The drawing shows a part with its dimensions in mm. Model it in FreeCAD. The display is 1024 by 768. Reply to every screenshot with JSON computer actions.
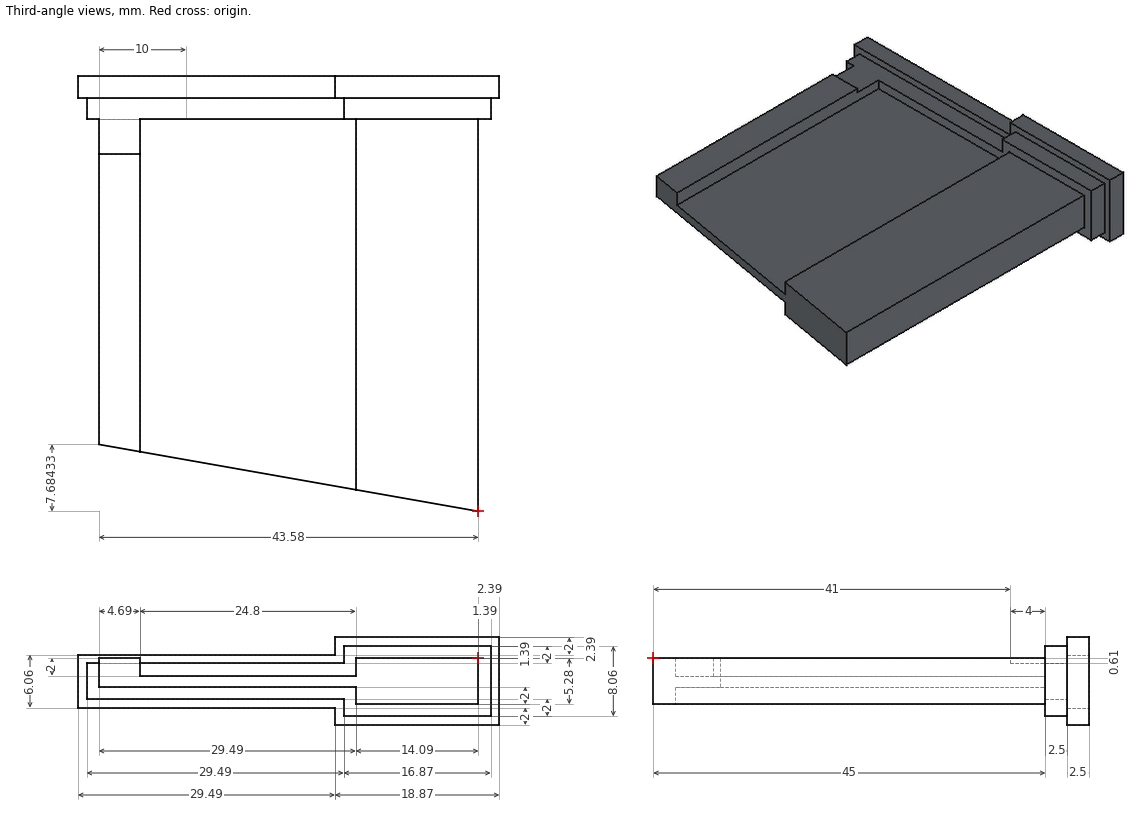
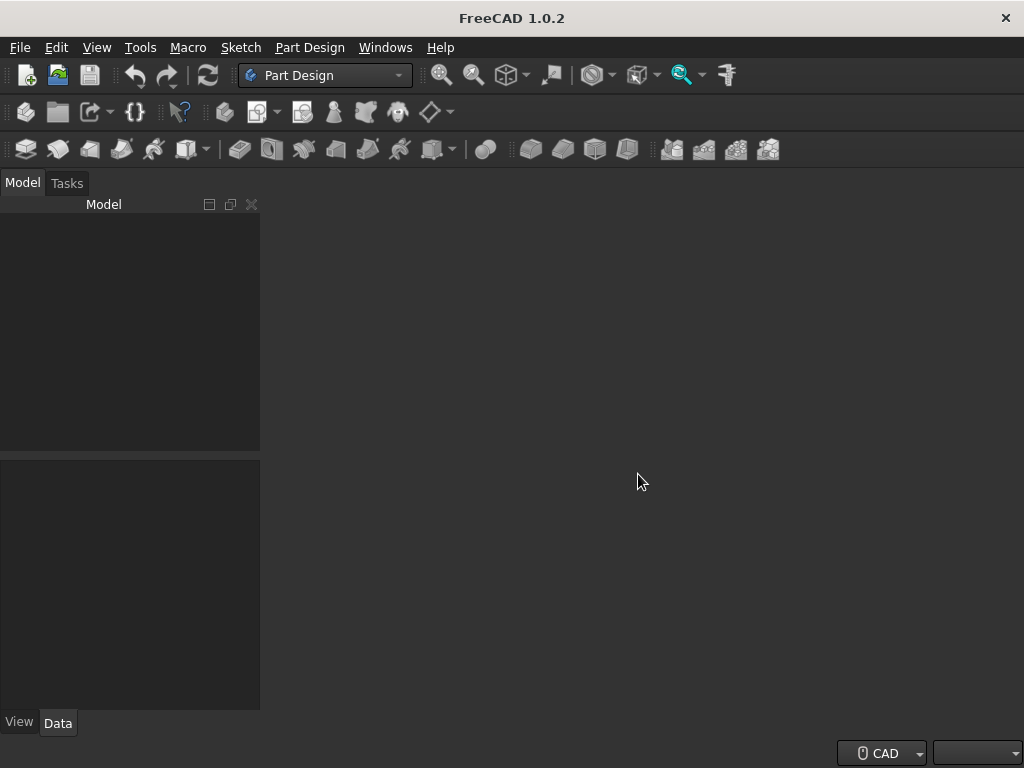
{"action": "left_click", "coordinate": [26, 76]}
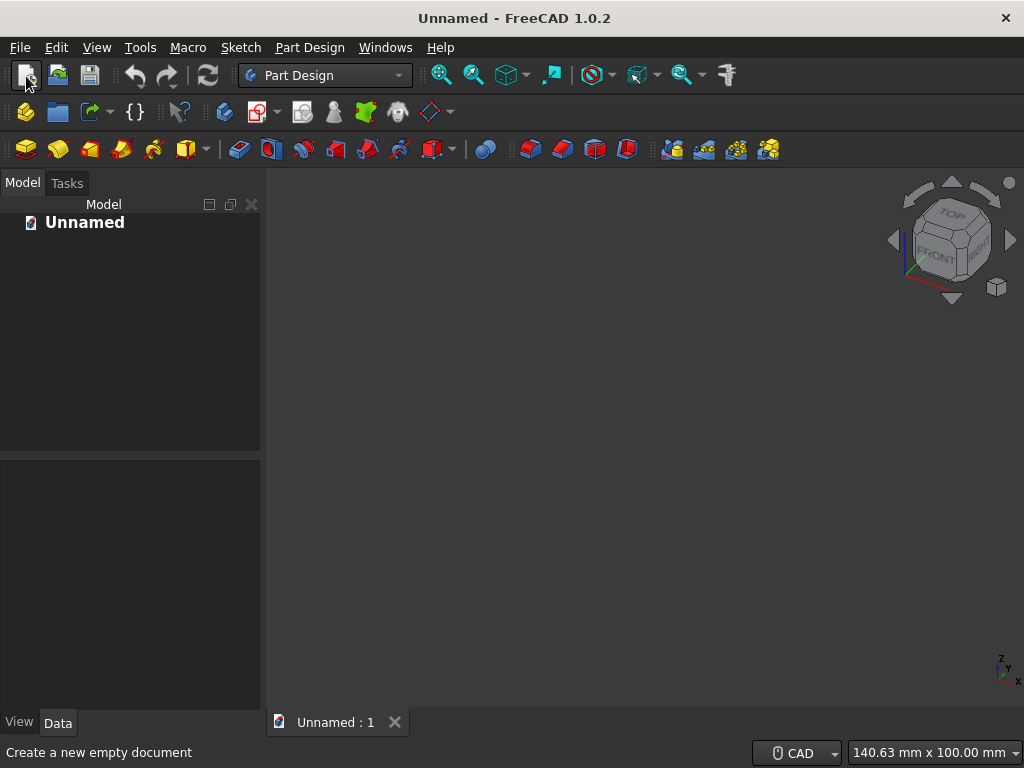
{"action": "left_click", "coordinate": [258, 112]}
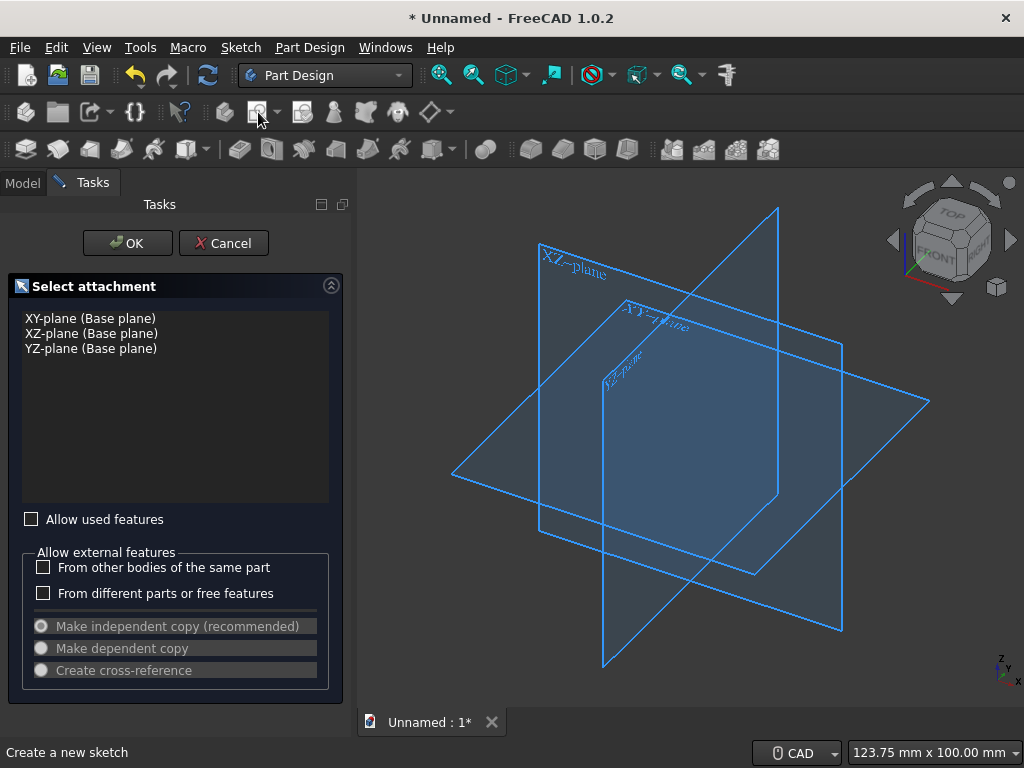
{"action": "left_click", "coordinate": [82, 334]}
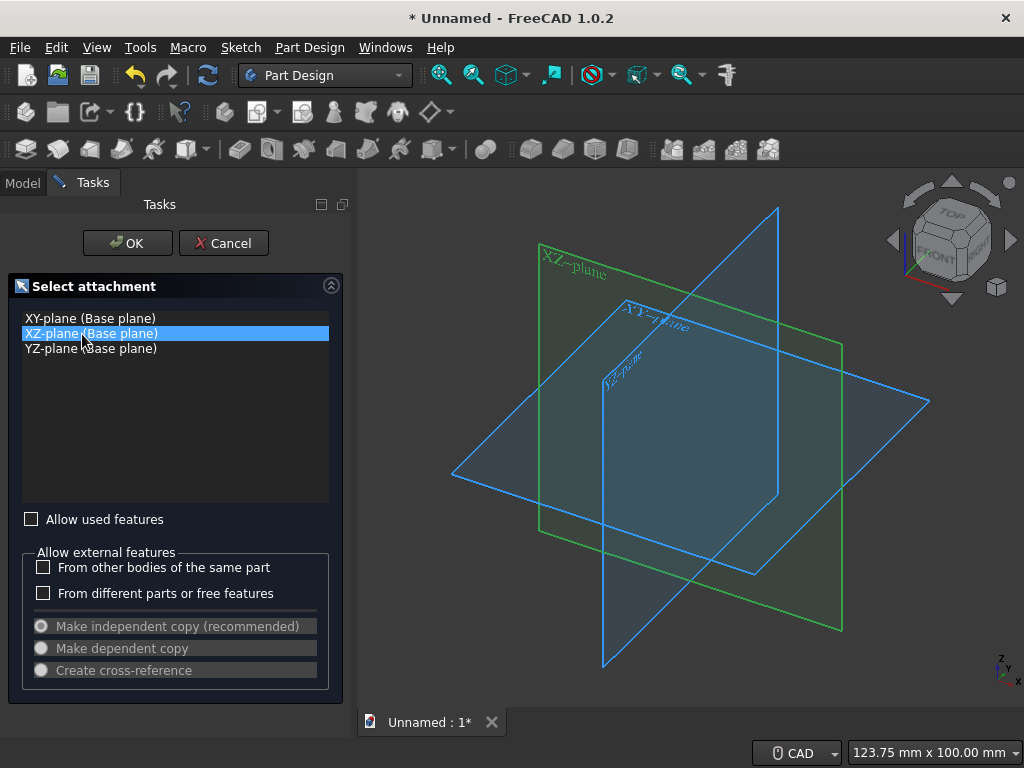
{"action": "left_click", "coordinate": [128, 243]}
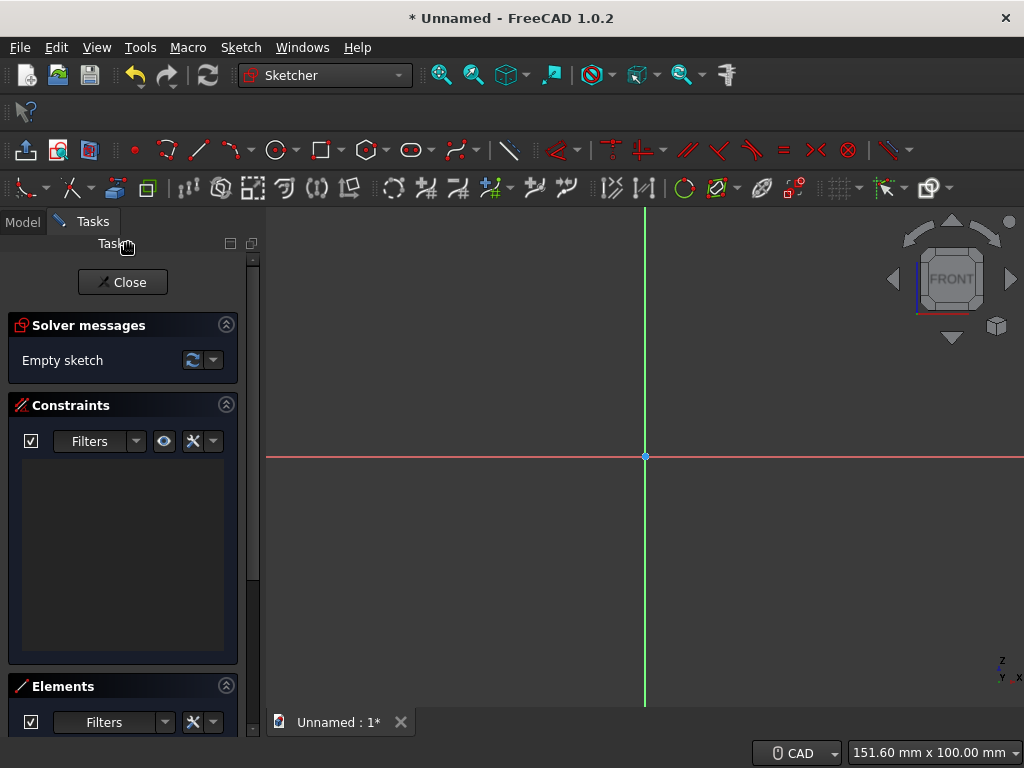
{"action": "scroll", "coordinate": [487, 486], "scroll_direction": "up", "scroll_amount": 3}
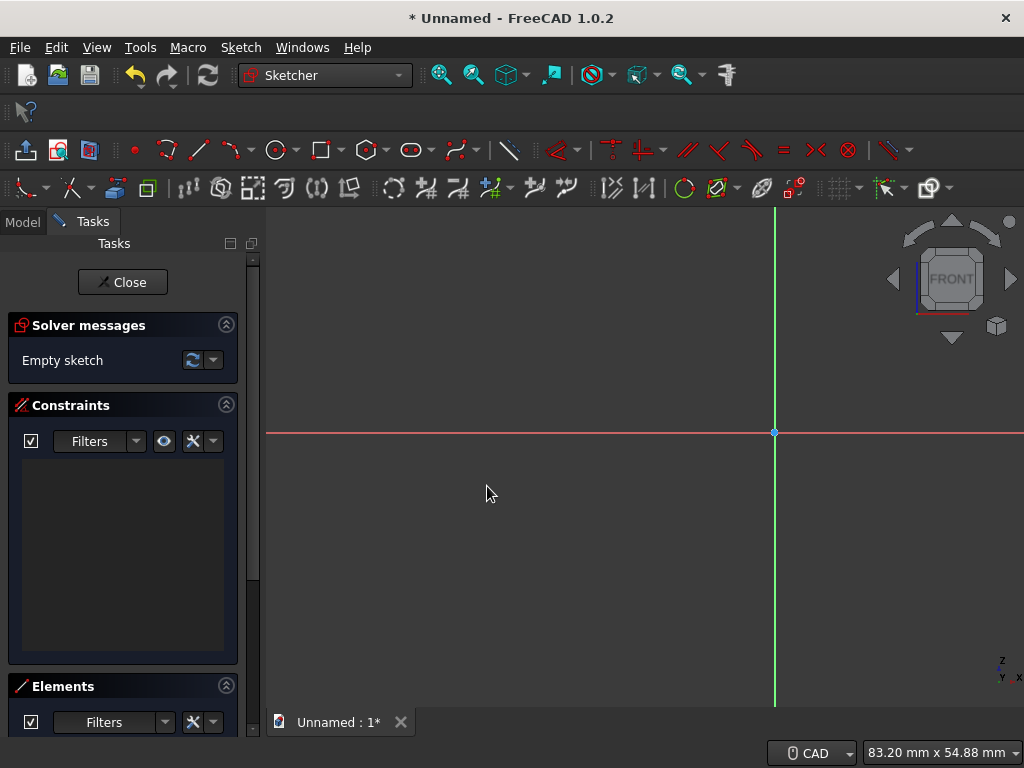
{"action": "left_click", "coordinate": [168, 150]}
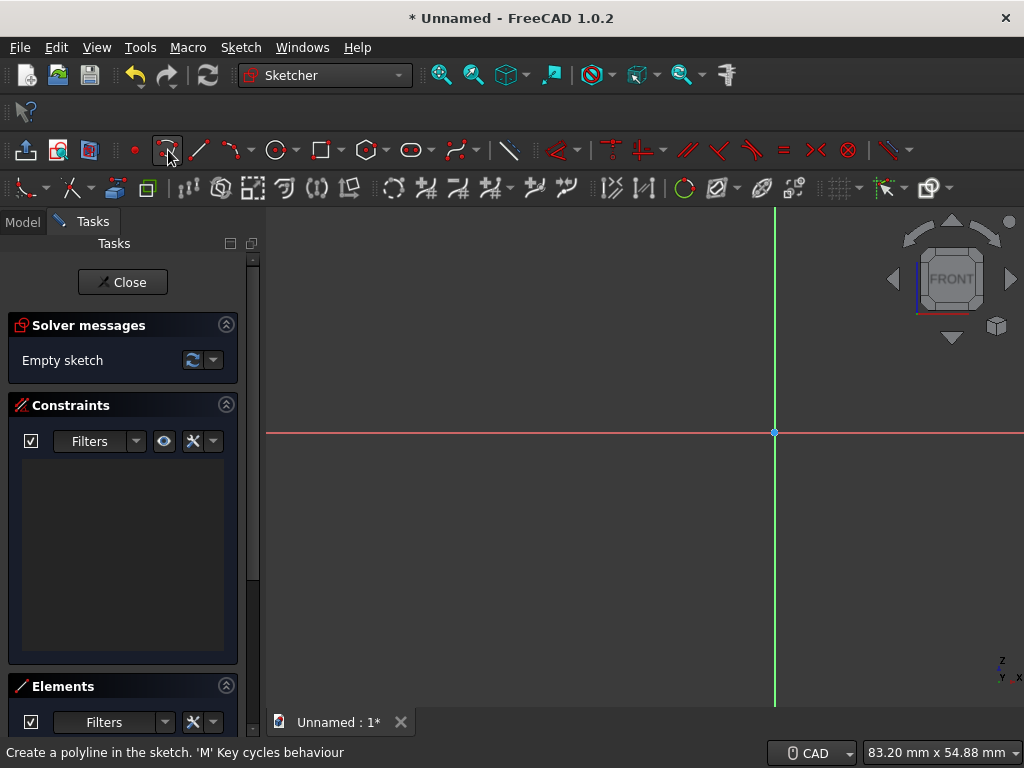
{"action": "left_click", "coordinate": [775, 433]}
{"action": "left_click", "coordinate": [766, 481]}
{"action": "left_click", "coordinate": [646, 481]}
{"action": "left_click", "coordinate": [646, 463]}
{"action": "left_click", "coordinate": [378, 463]}
{"action": "left_click", "coordinate": [378, 433]}
{"action": "left_click", "coordinate": [420, 442]}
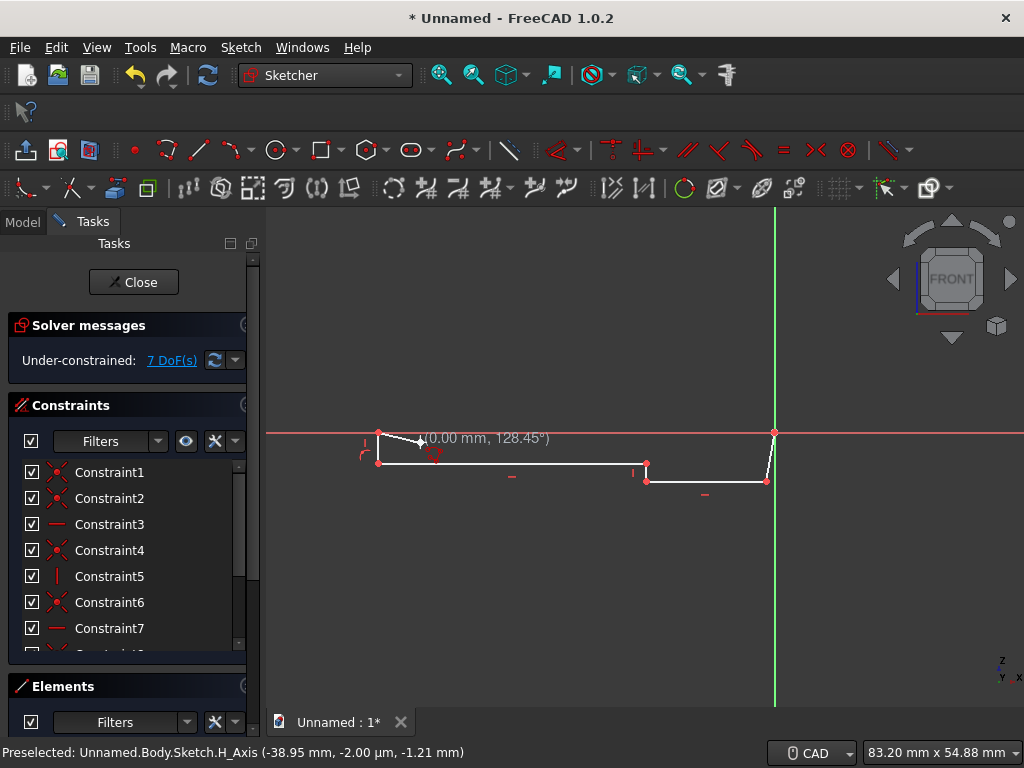
{"action": "scroll", "coordinate": [420, 451], "scroll_direction": "up", "scroll_amount": 2}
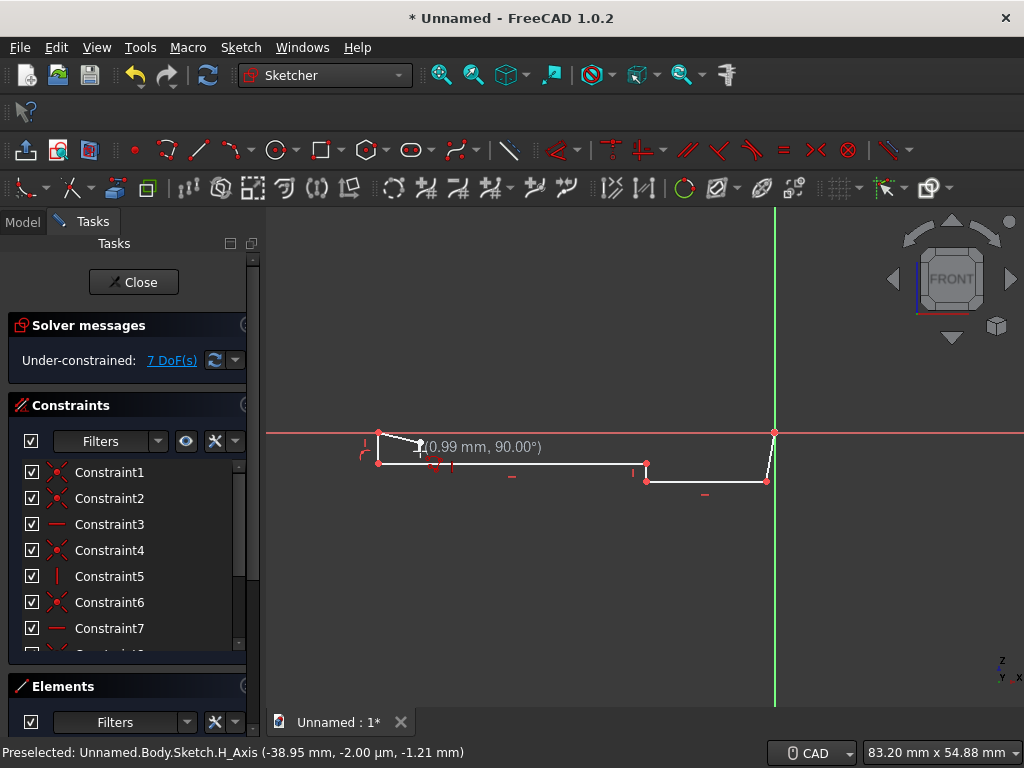
{"action": "left_click", "coordinate": [420, 451]}
{"action": "left_click", "coordinate": [757, 451]}
{"action": "left_click", "coordinate": [757, 432]}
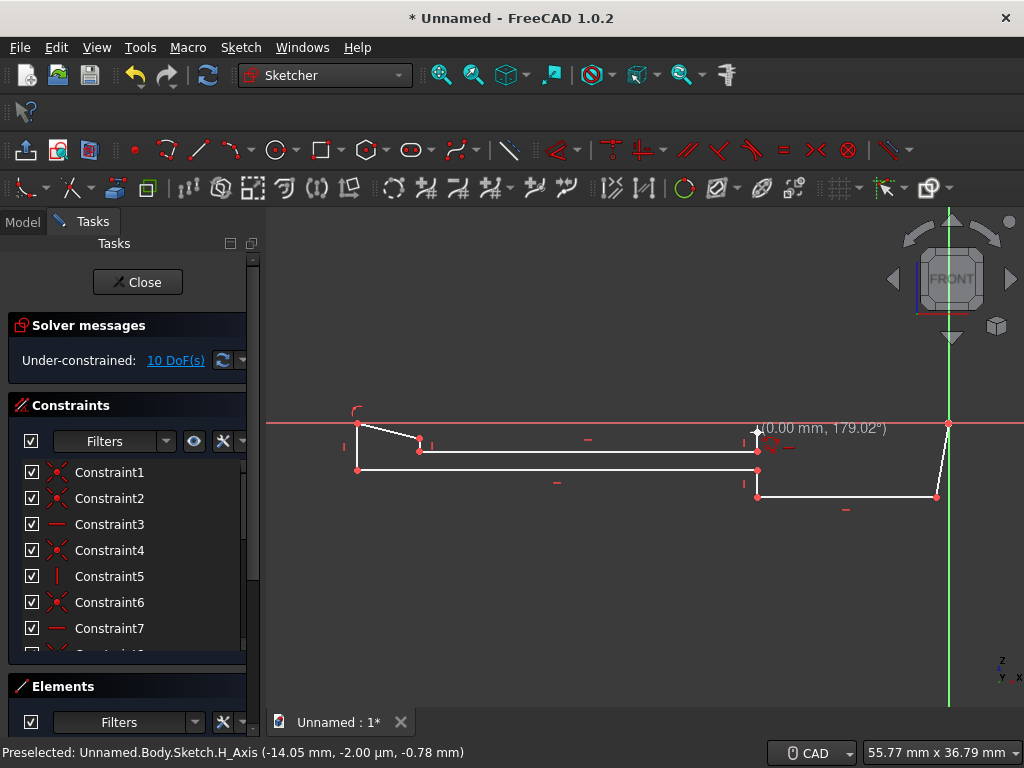
{"action": "scroll", "coordinate": [421, 452], "scroll_direction": "down", "scroll_amount": 2}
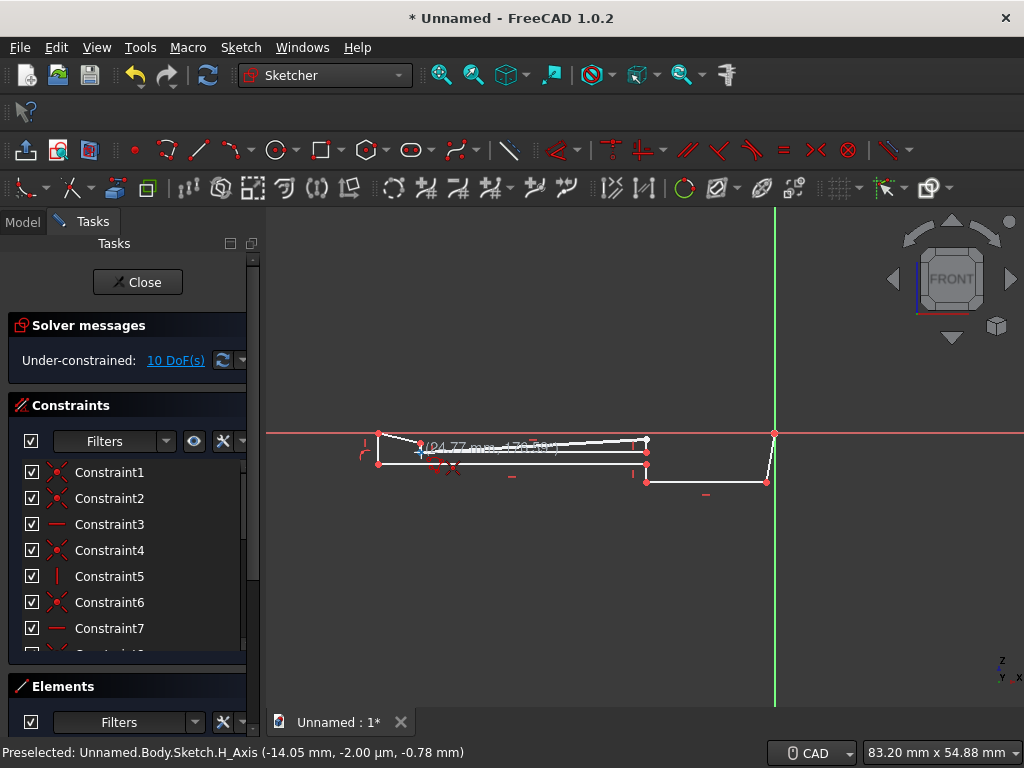
{"action": "left_click", "coordinate": [775, 433]}
{"action": "key", "text": "Escape"}
{"action": "key", "text": "Escape"}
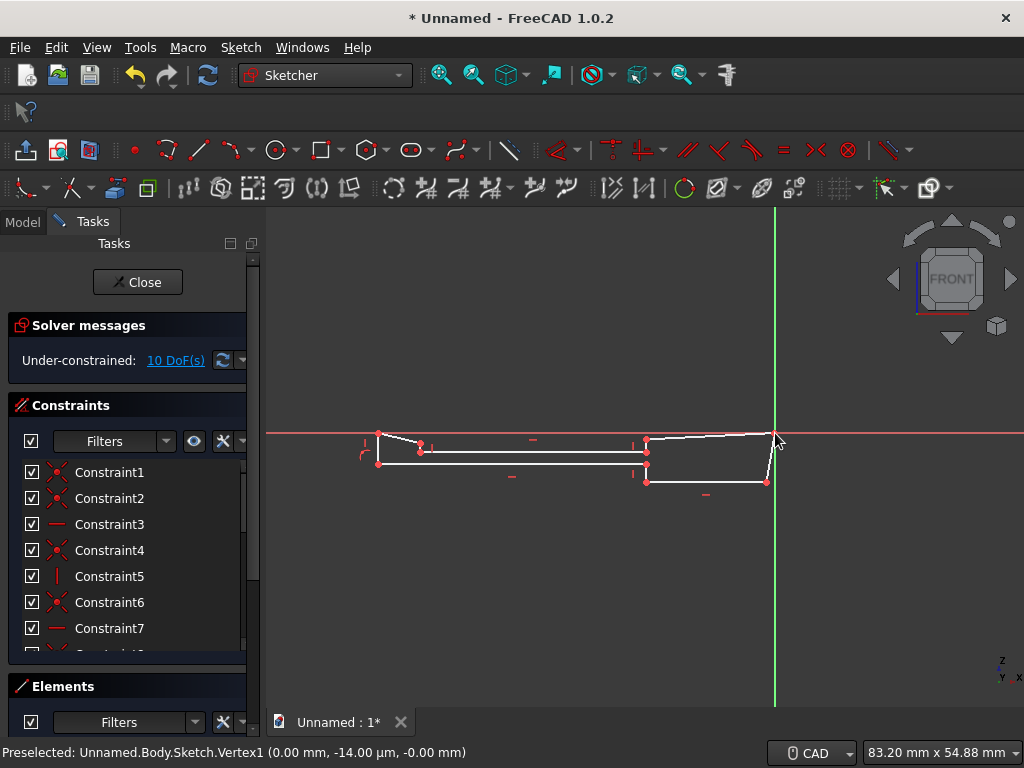
{"action": "left_click", "coordinate": [772, 448]}